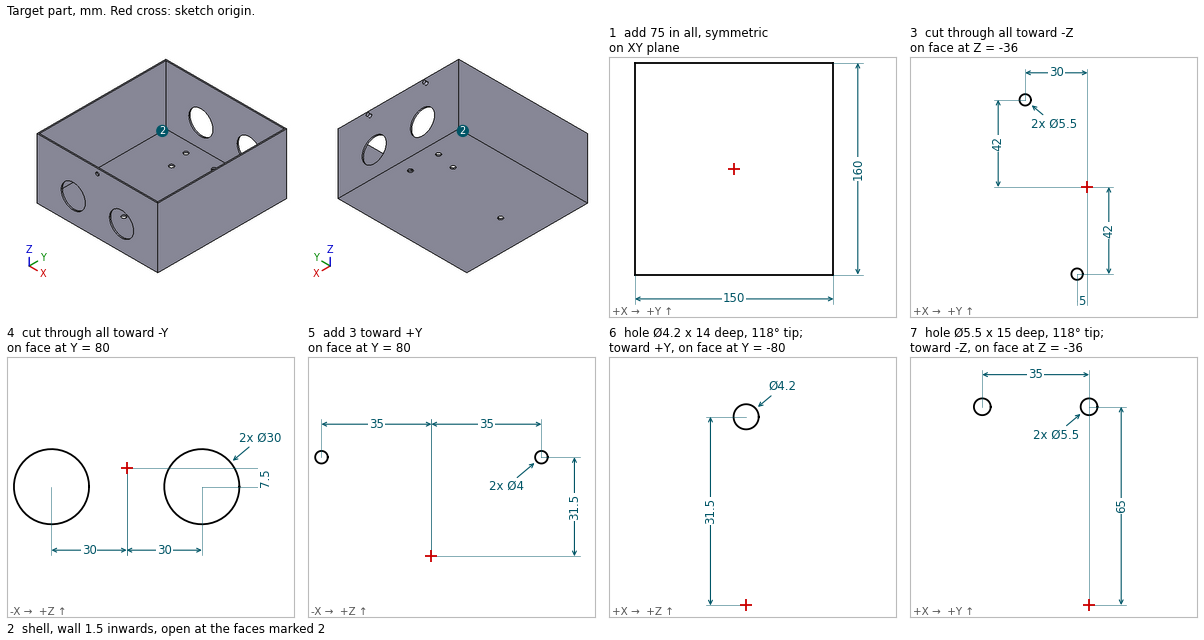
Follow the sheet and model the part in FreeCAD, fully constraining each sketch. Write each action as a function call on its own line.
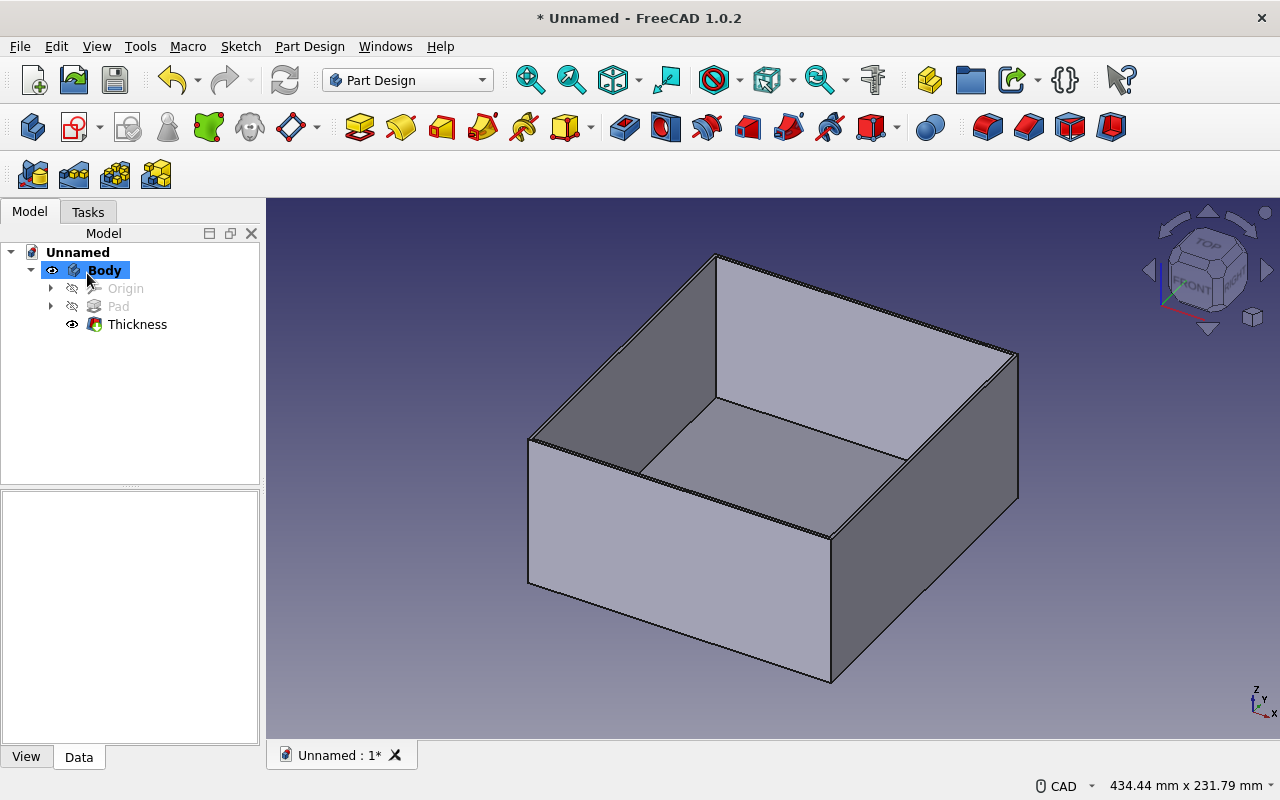
click(799, 510)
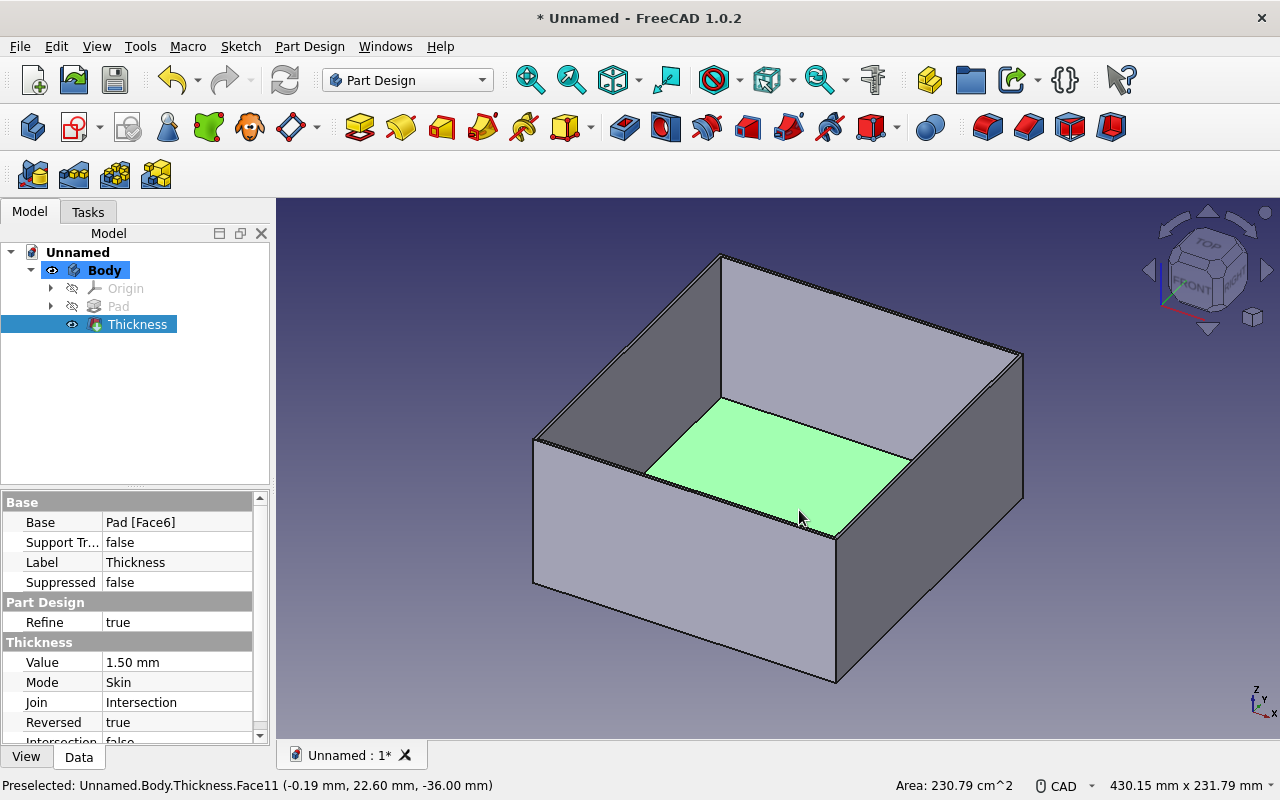
click(74, 128)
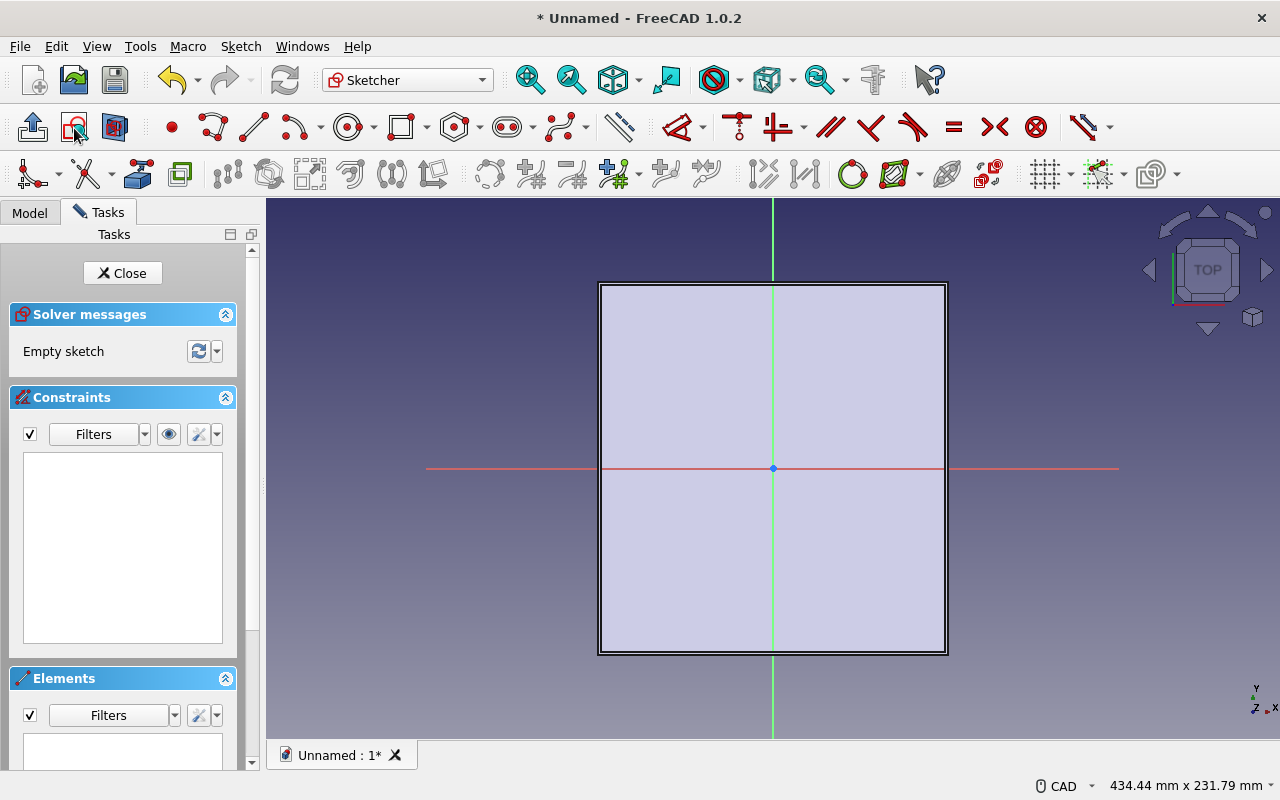
key(q)
key(s)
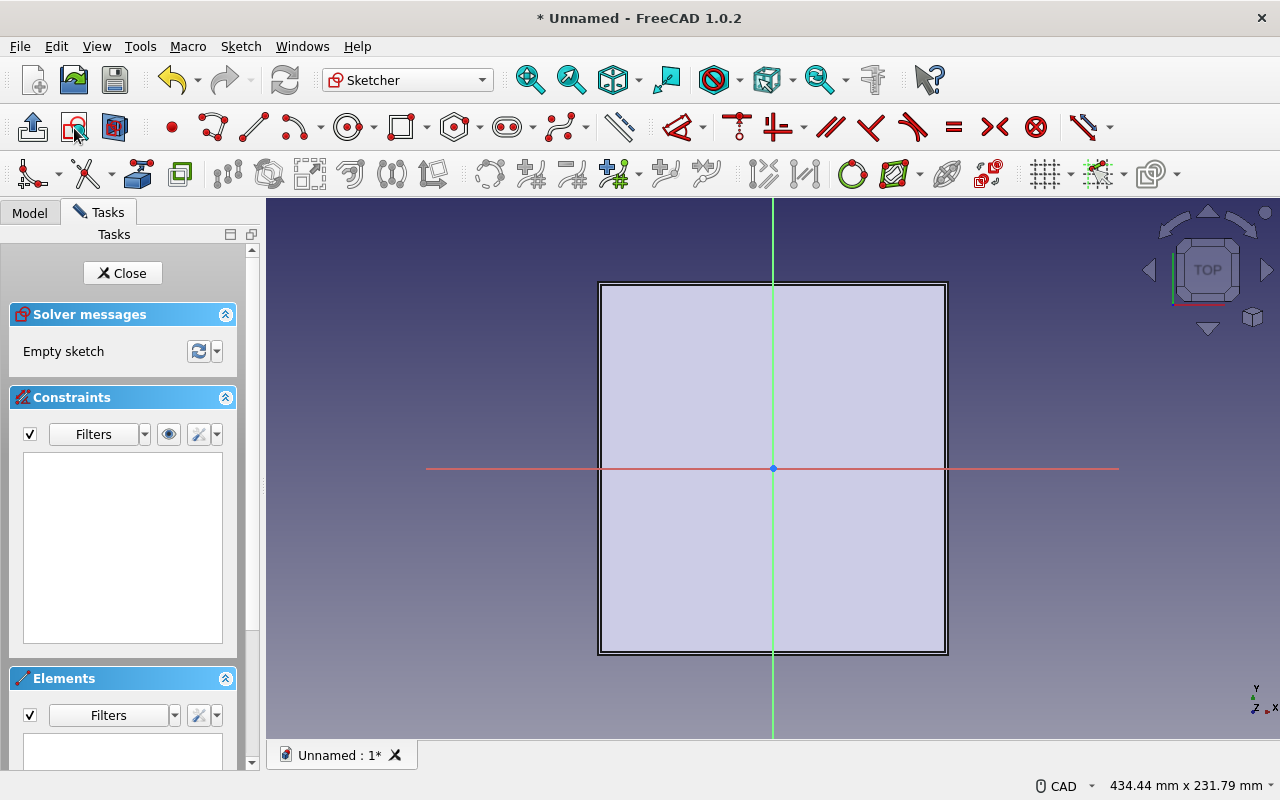
scroll(796, 469, up, 2)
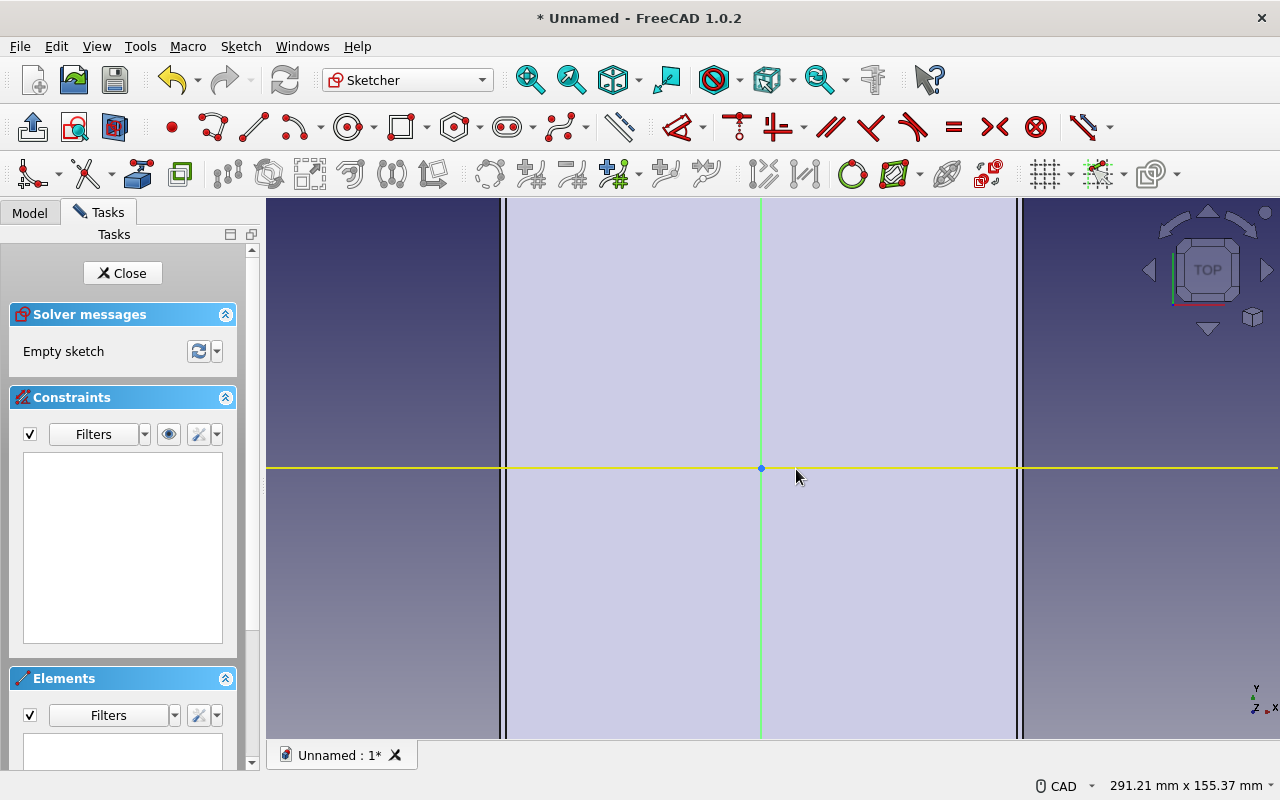
key(g)
key(c)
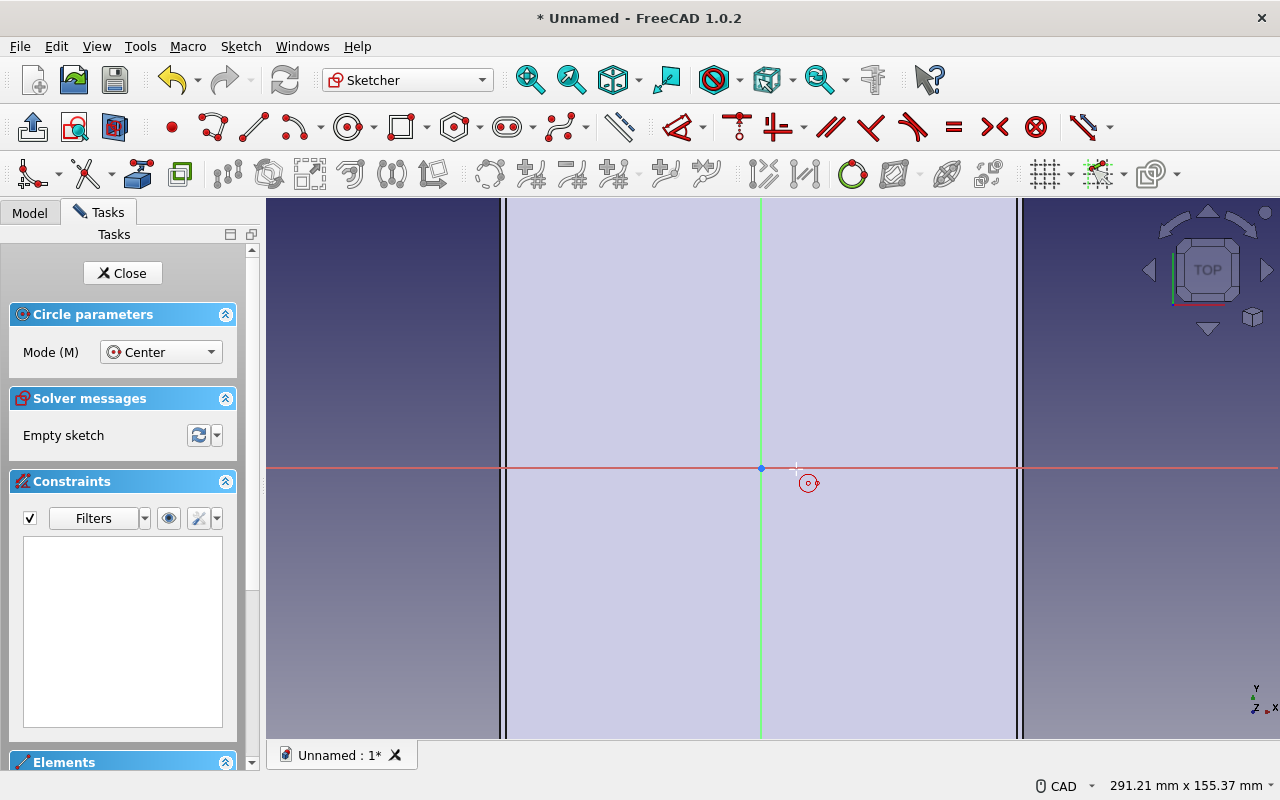
scroll(657, 322, up, 5)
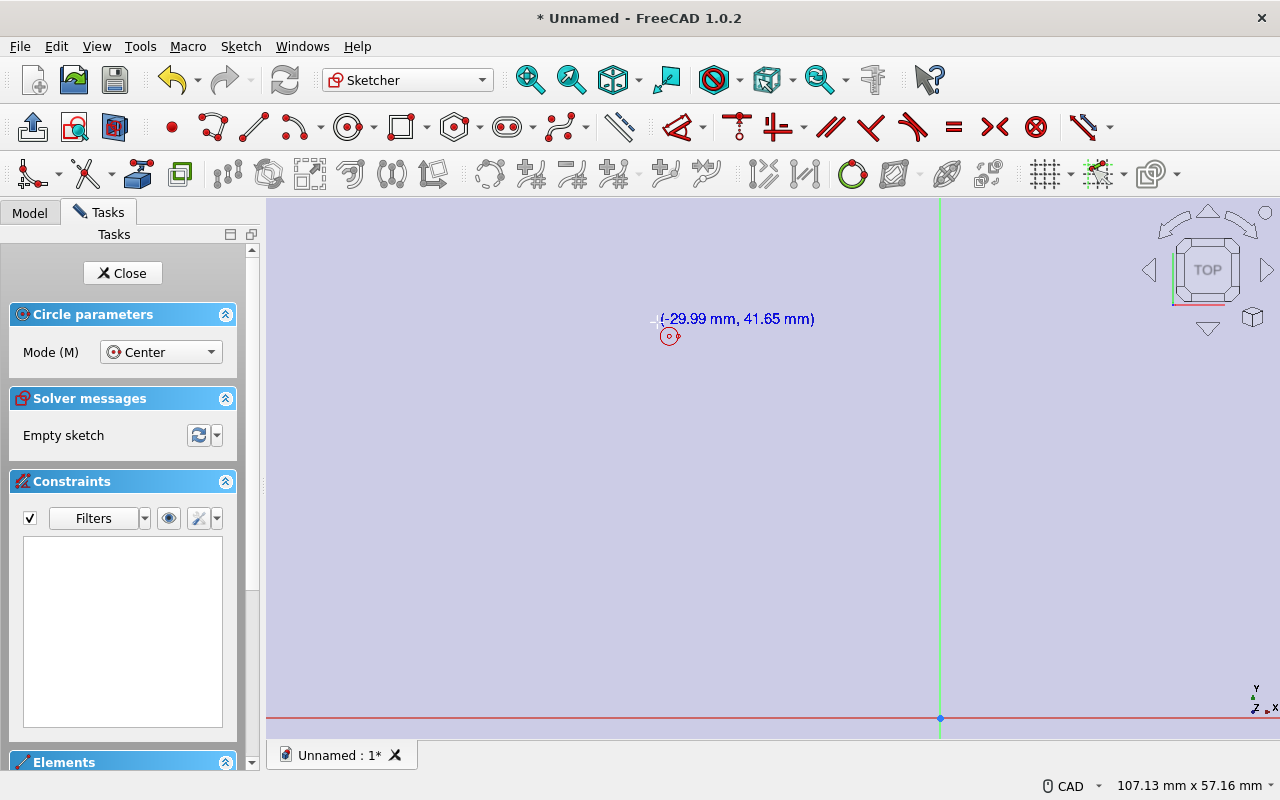
click(656, 321)
move(675, 303)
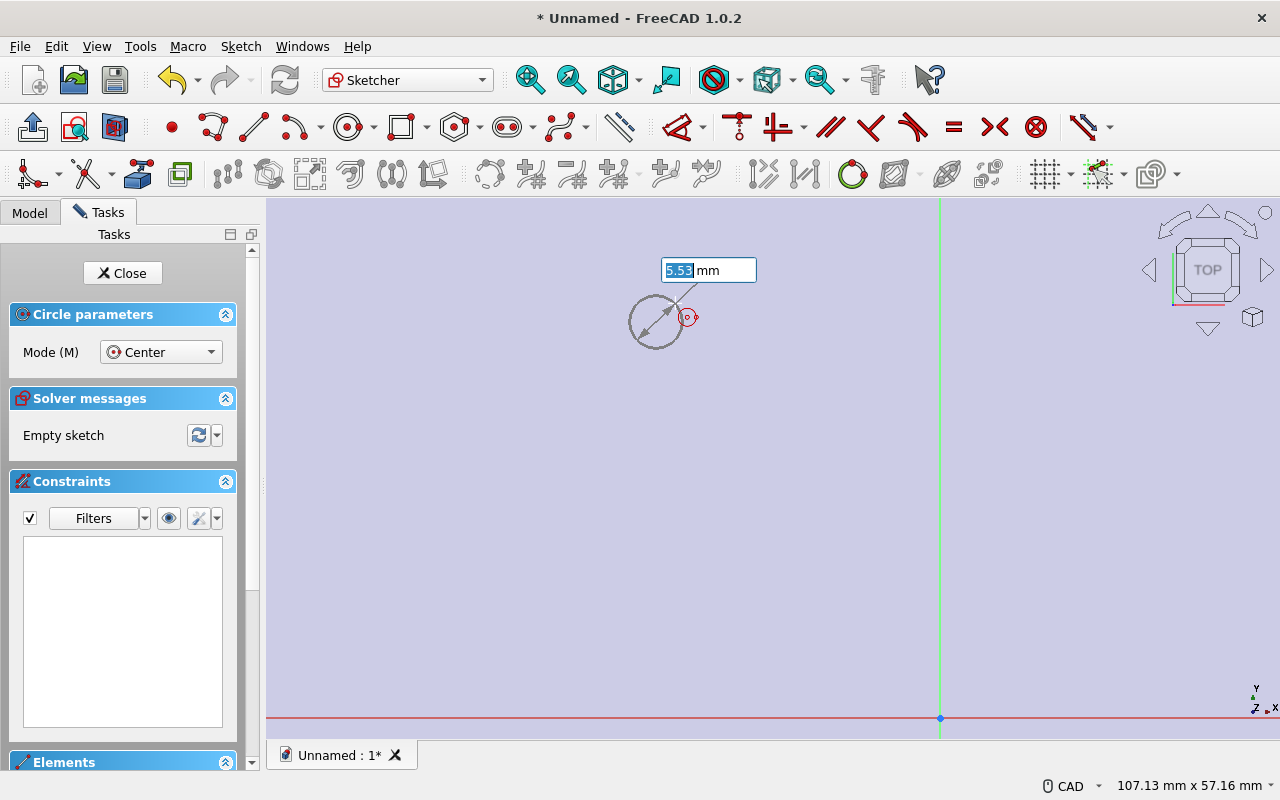
text(5.5)
key(Return)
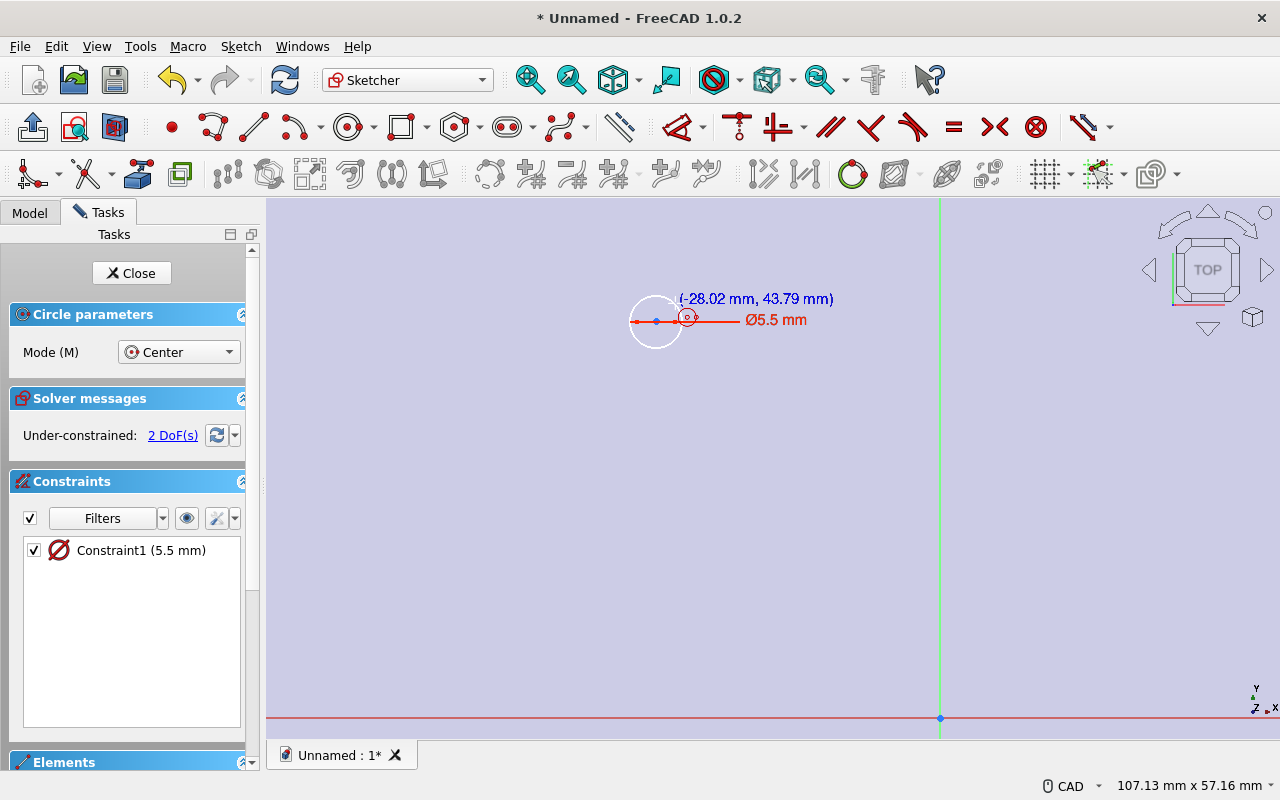
scroll(658, 323, down, 5)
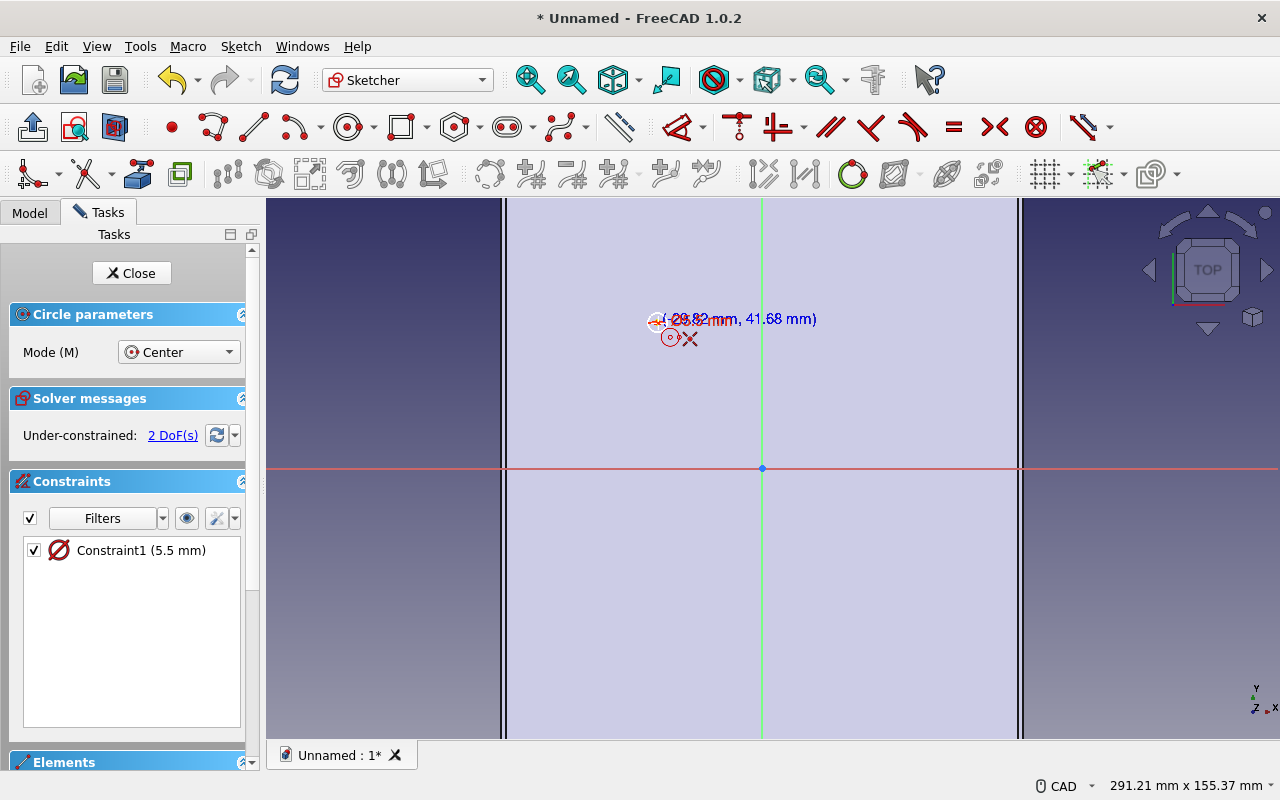
scroll(745, 615, up, 5)